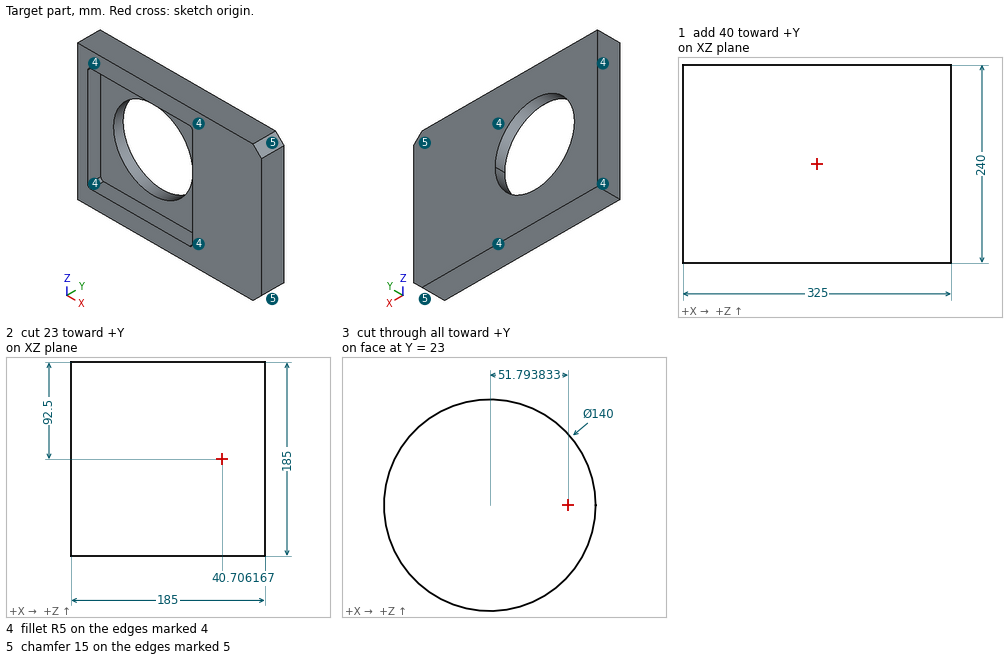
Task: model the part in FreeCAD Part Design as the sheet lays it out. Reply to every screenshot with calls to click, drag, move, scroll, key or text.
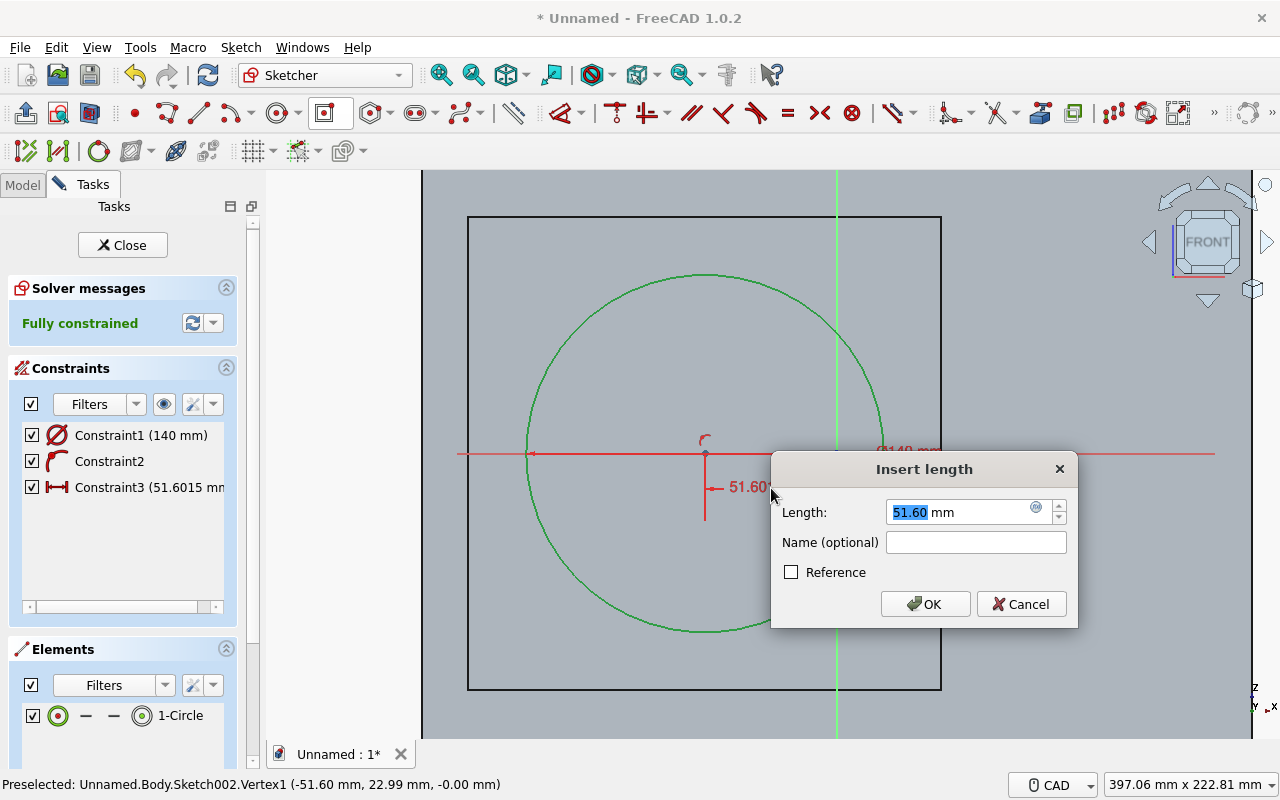
text(51.793833)
key(Return)
key(Escape)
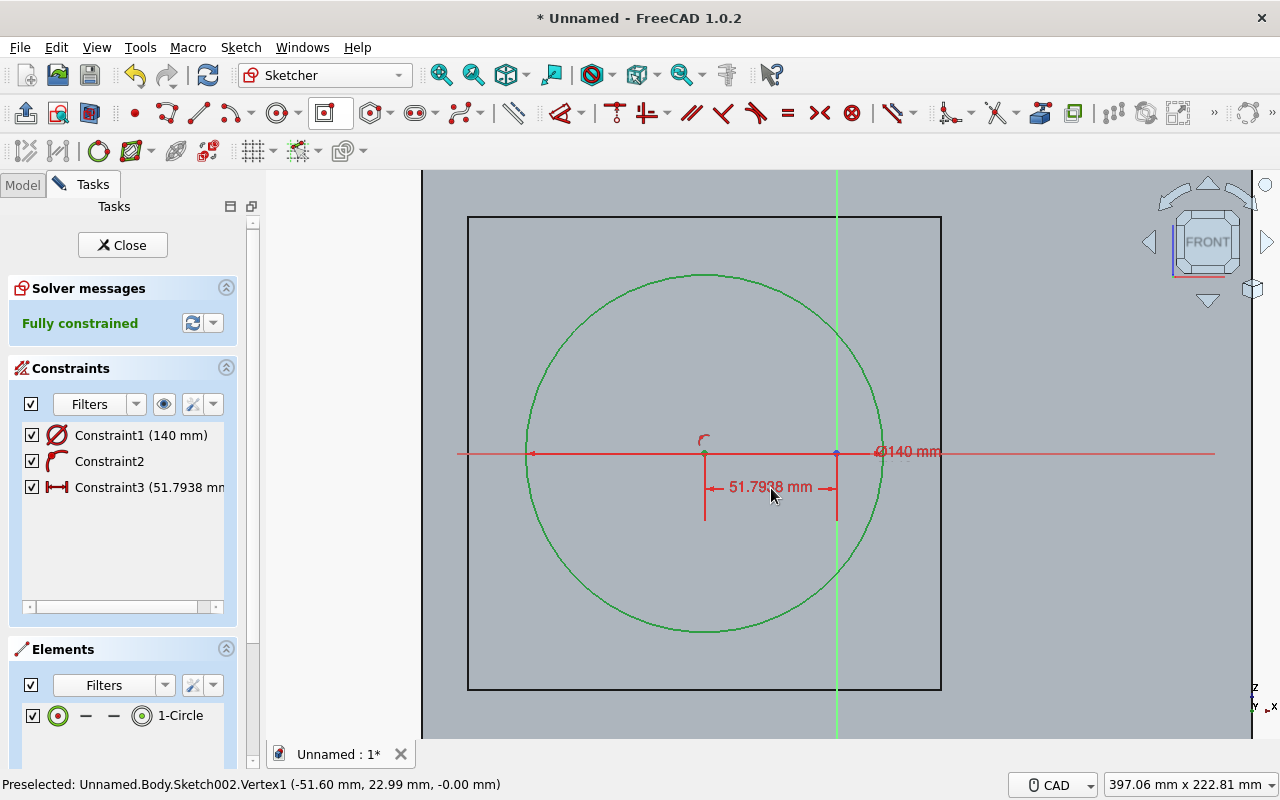
click(123, 245)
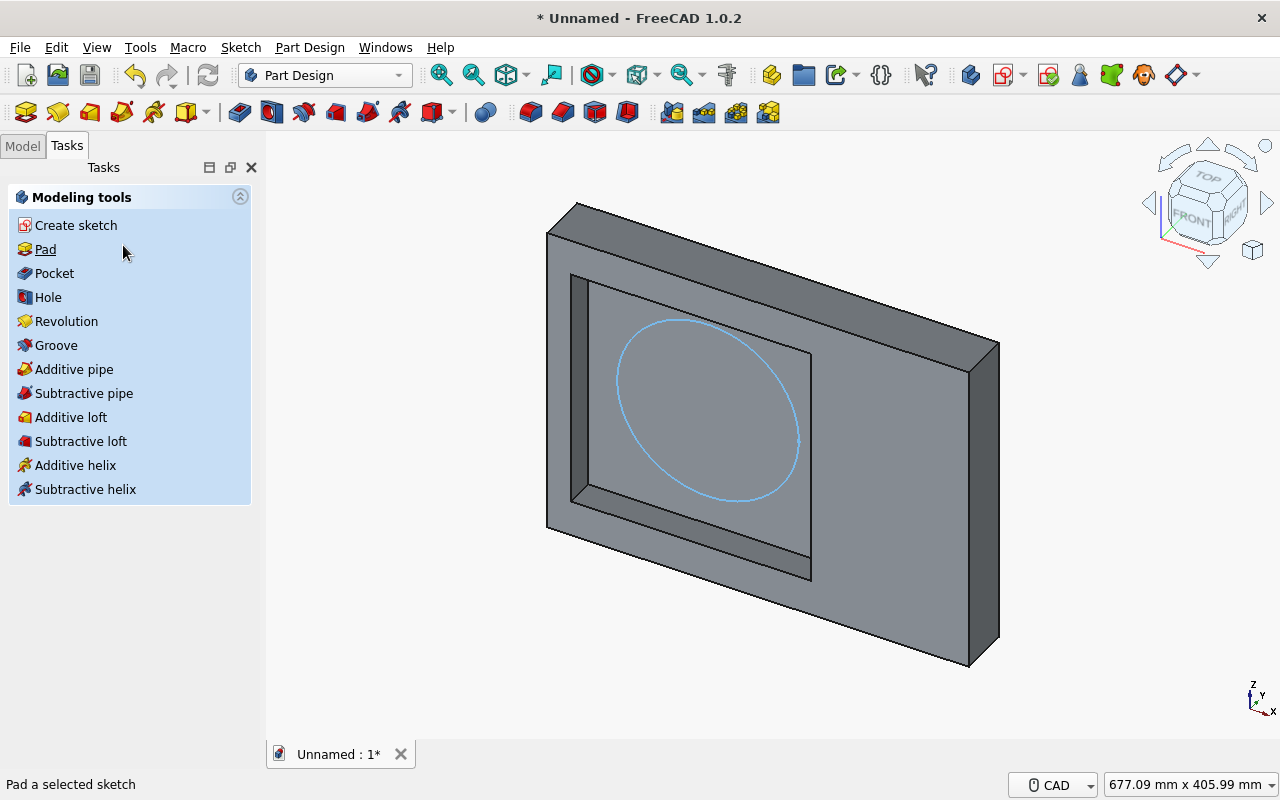
click(240, 112)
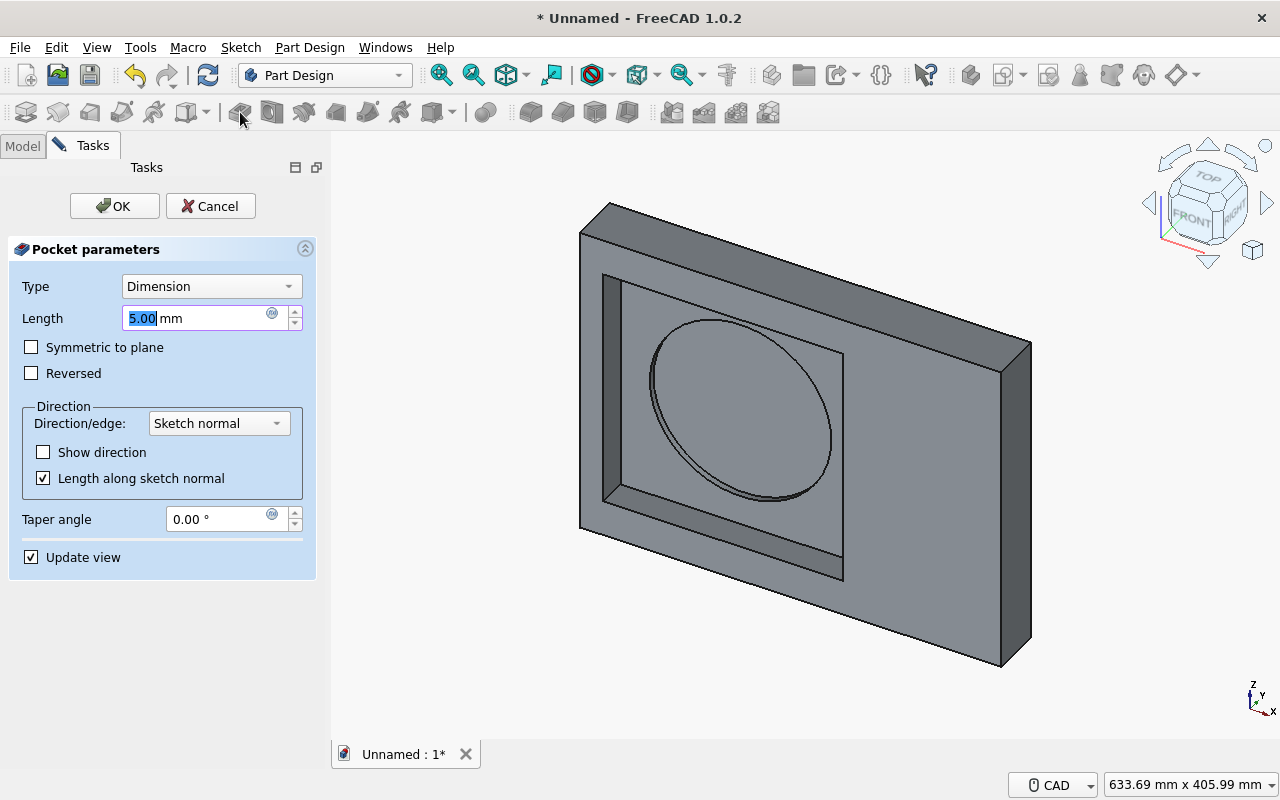
click(212, 286)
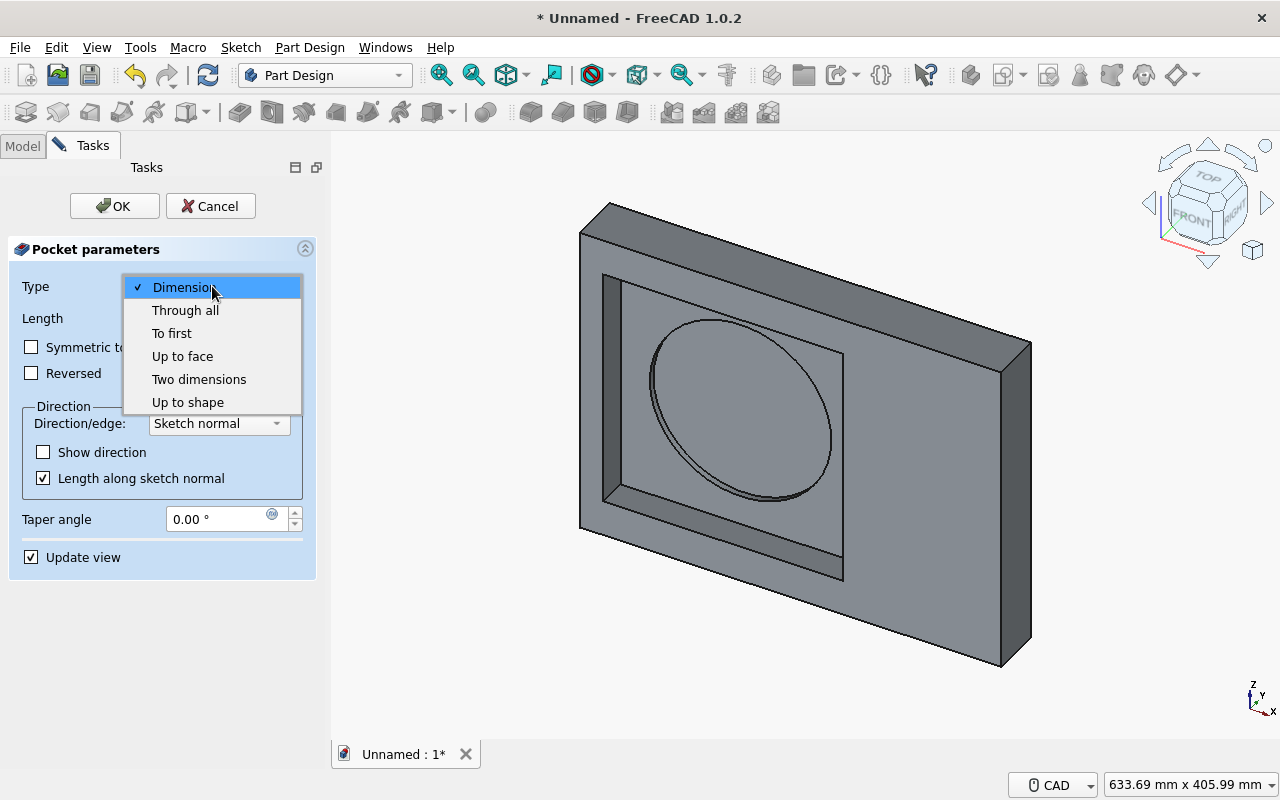
click(212, 310)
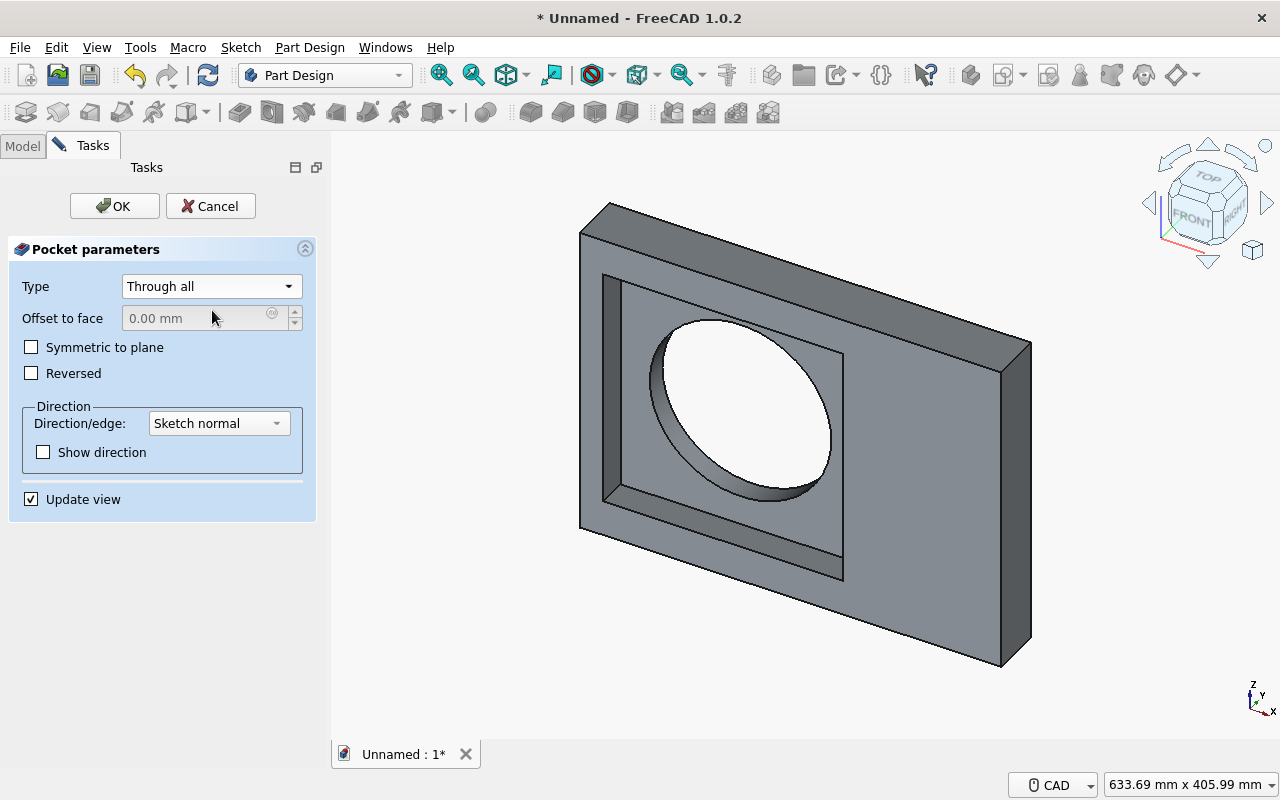
click(115, 206)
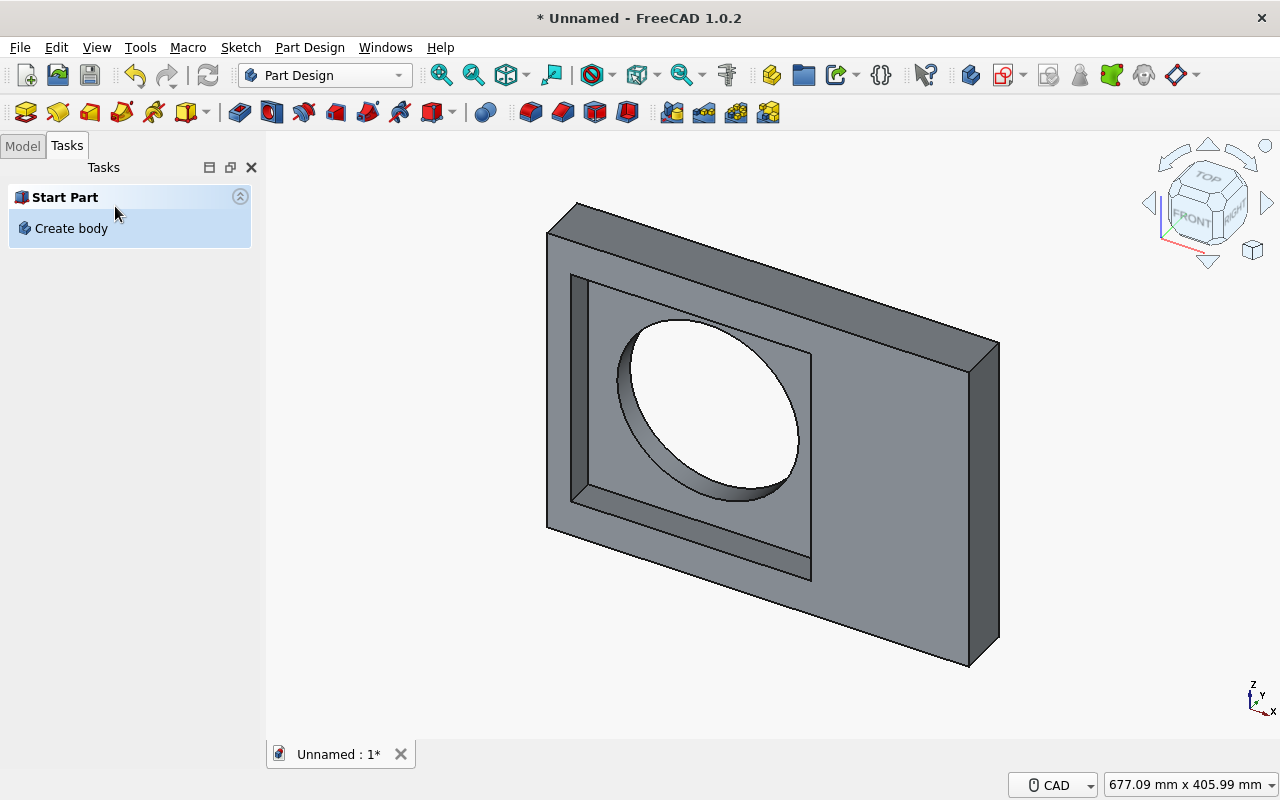
key(0)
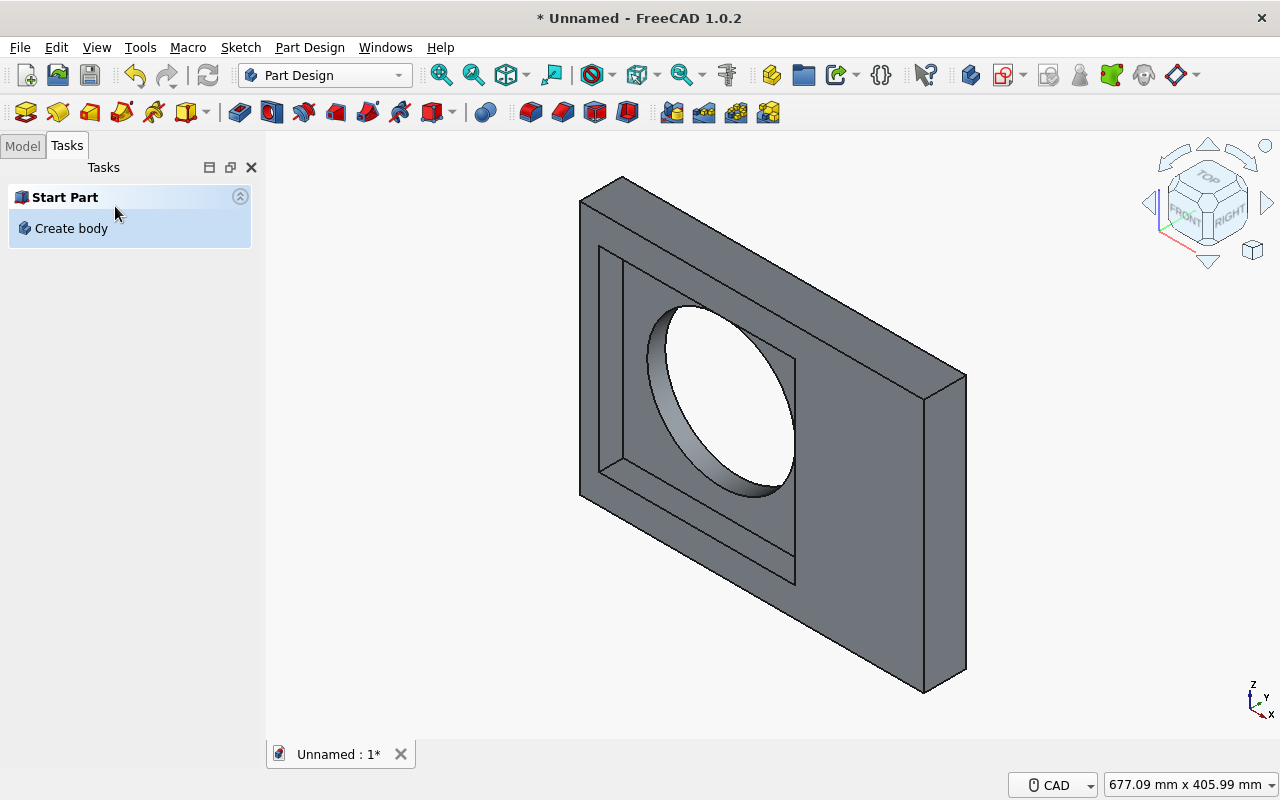
key(2)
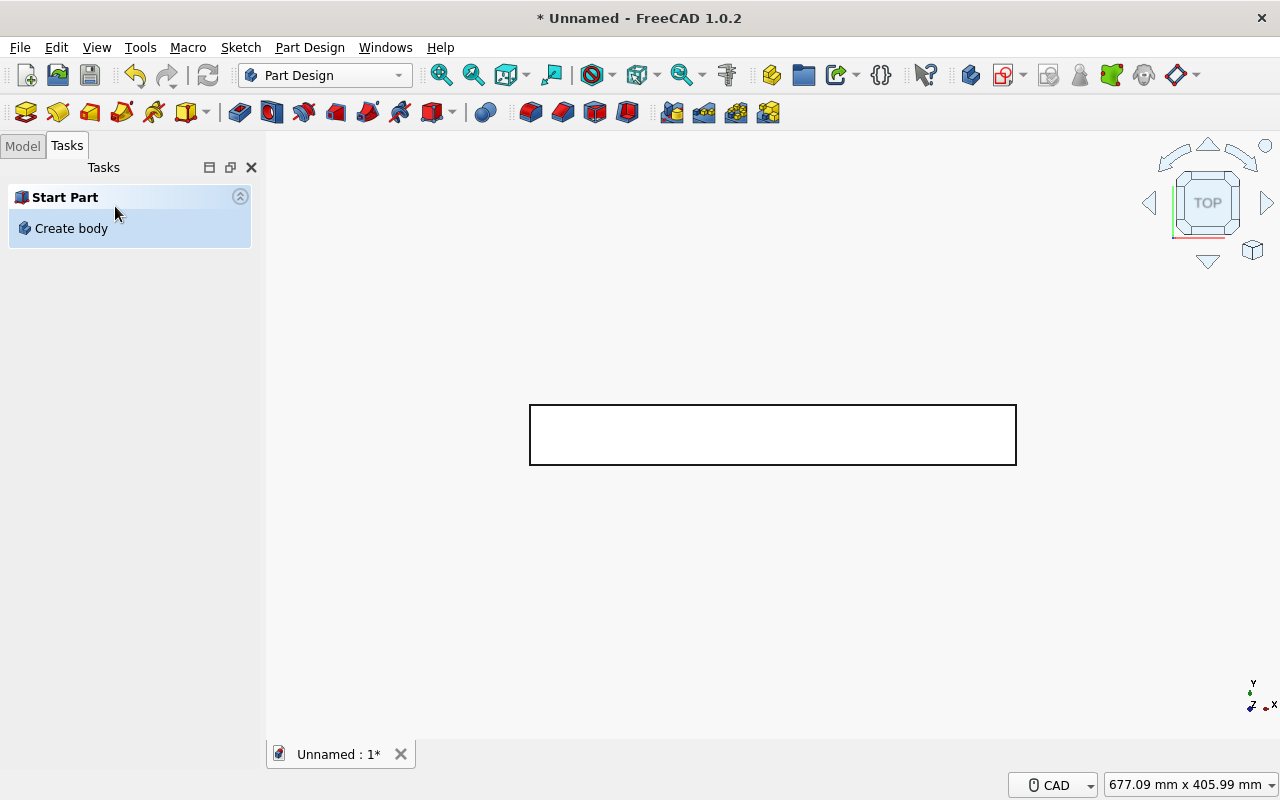
key(1)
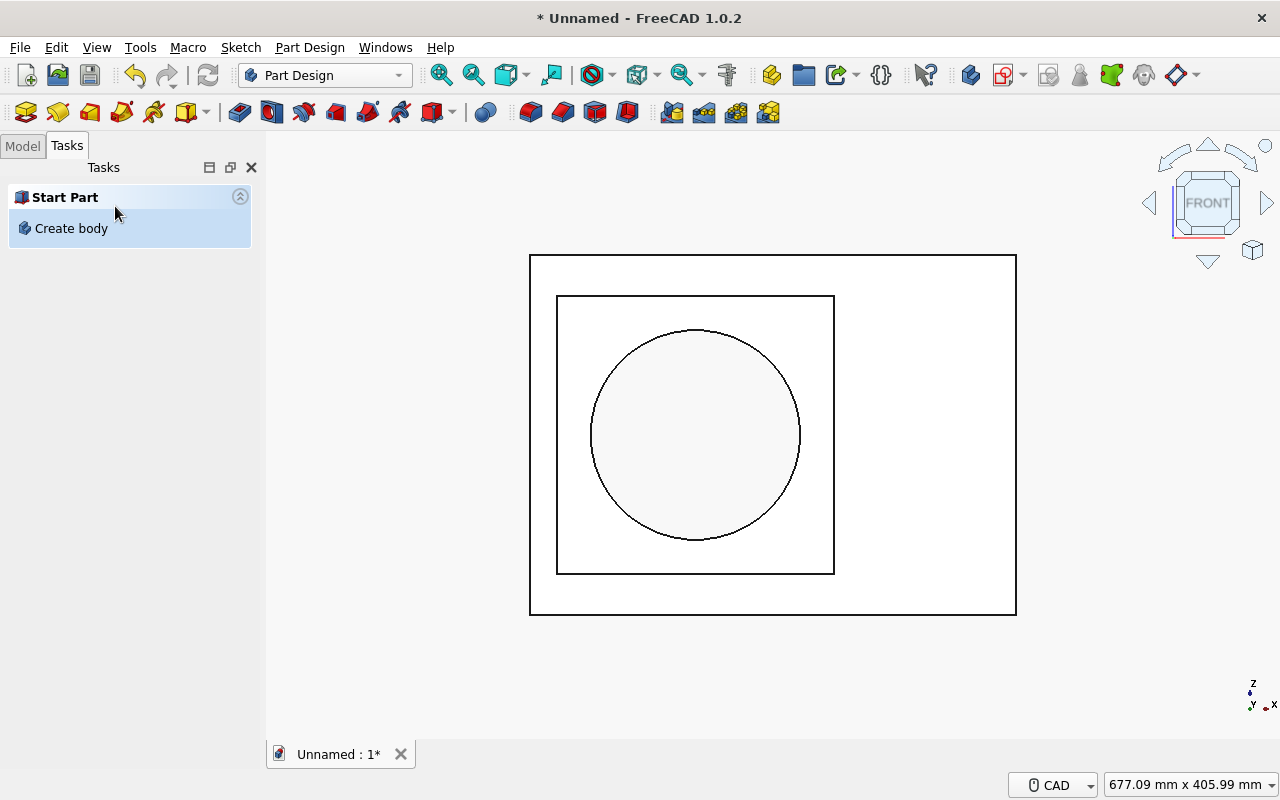
key(3)